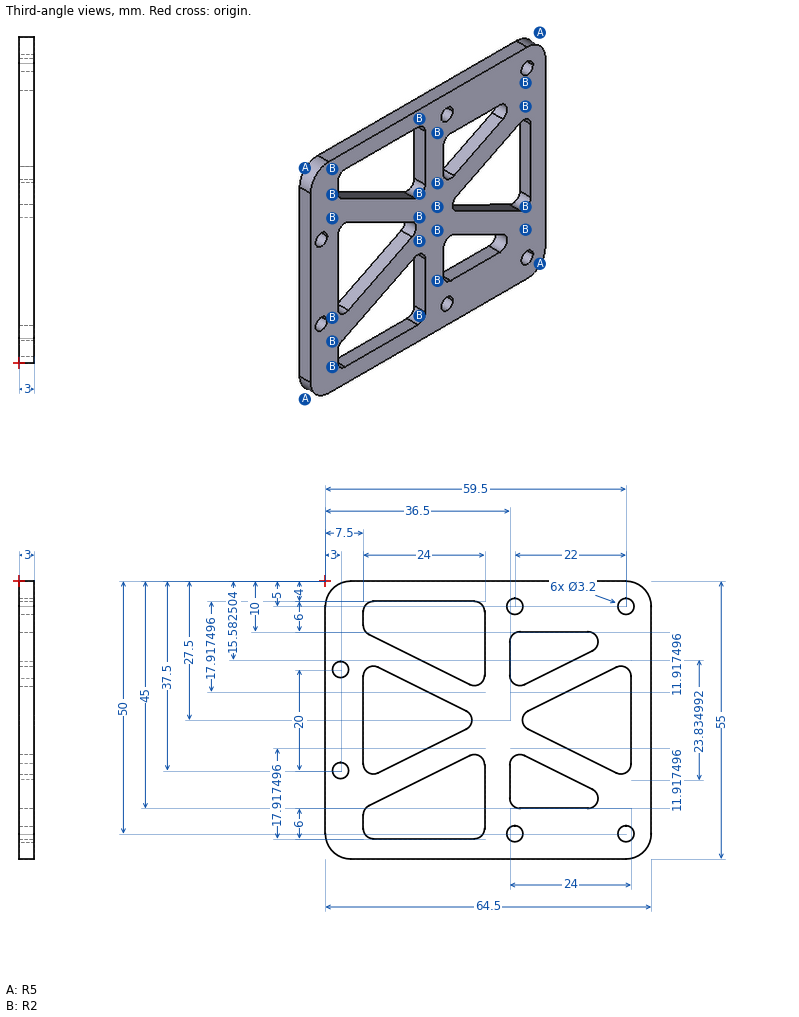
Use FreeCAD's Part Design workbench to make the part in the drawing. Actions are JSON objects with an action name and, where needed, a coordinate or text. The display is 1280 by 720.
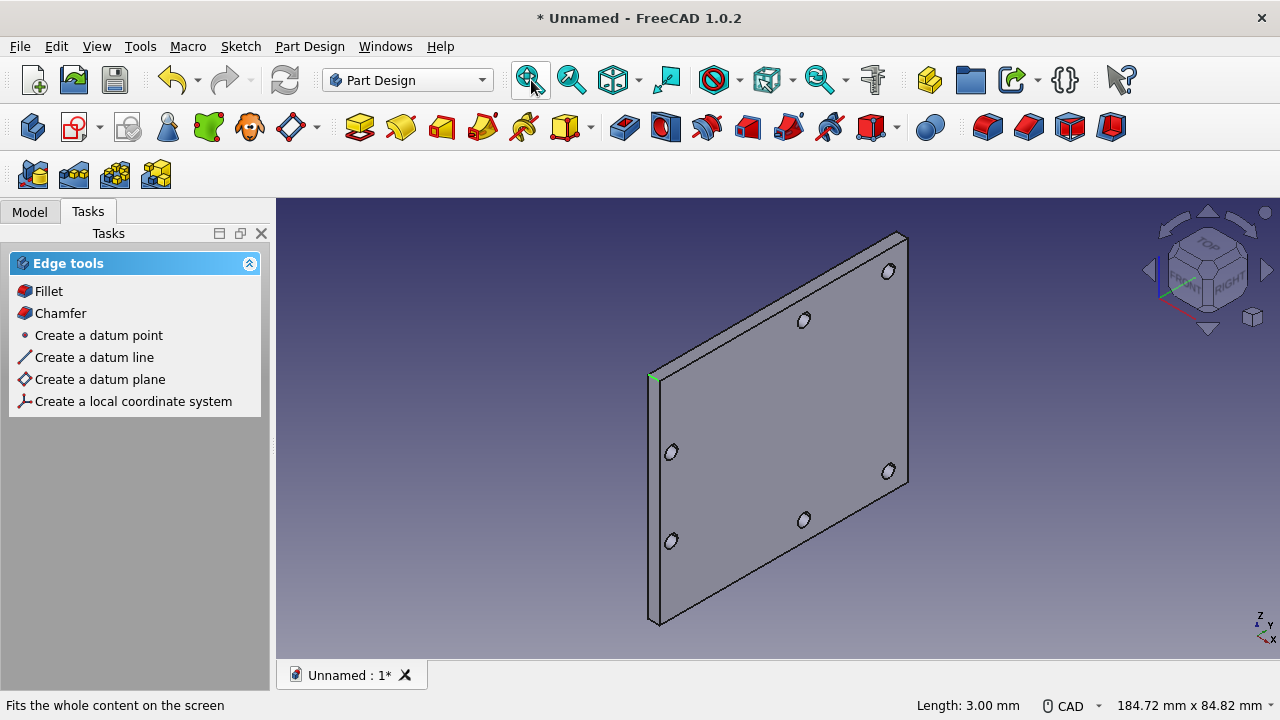
{"action": "scroll", "coordinate": [902, 234], "scroll_direction": "up", "scroll_amount": 5}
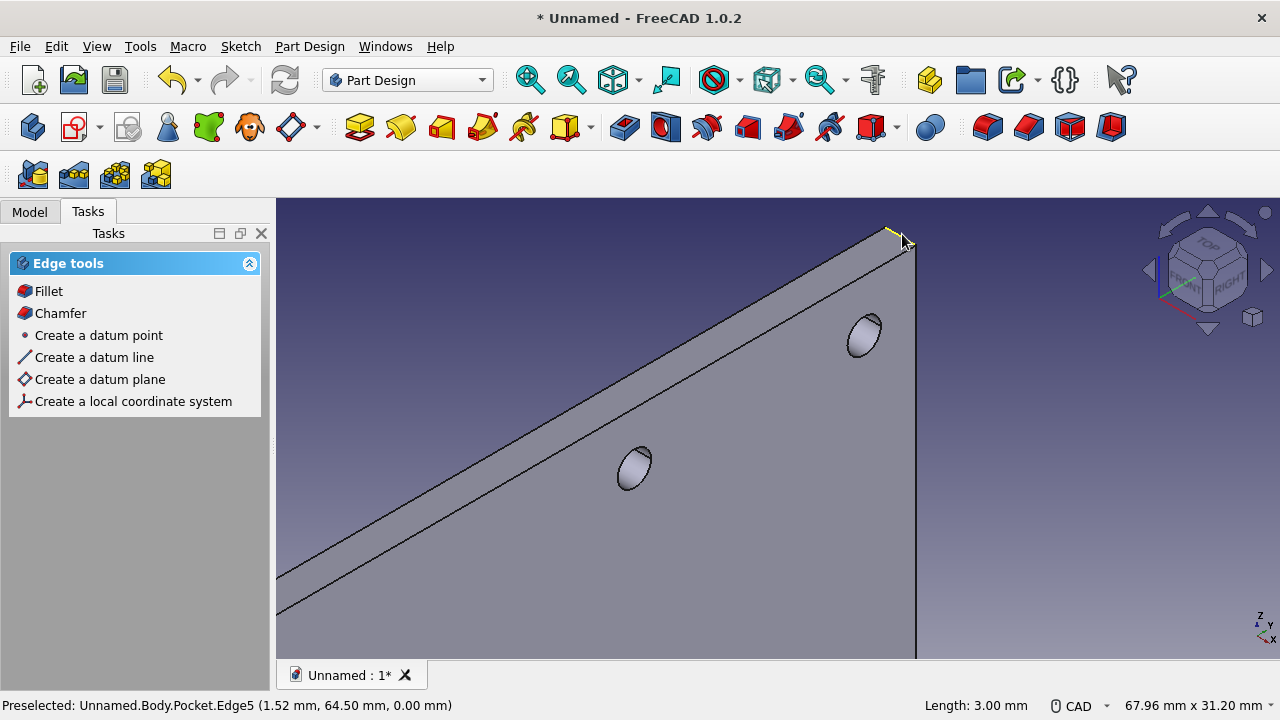
{"action": "left_click", "coordinate": [531, 80]}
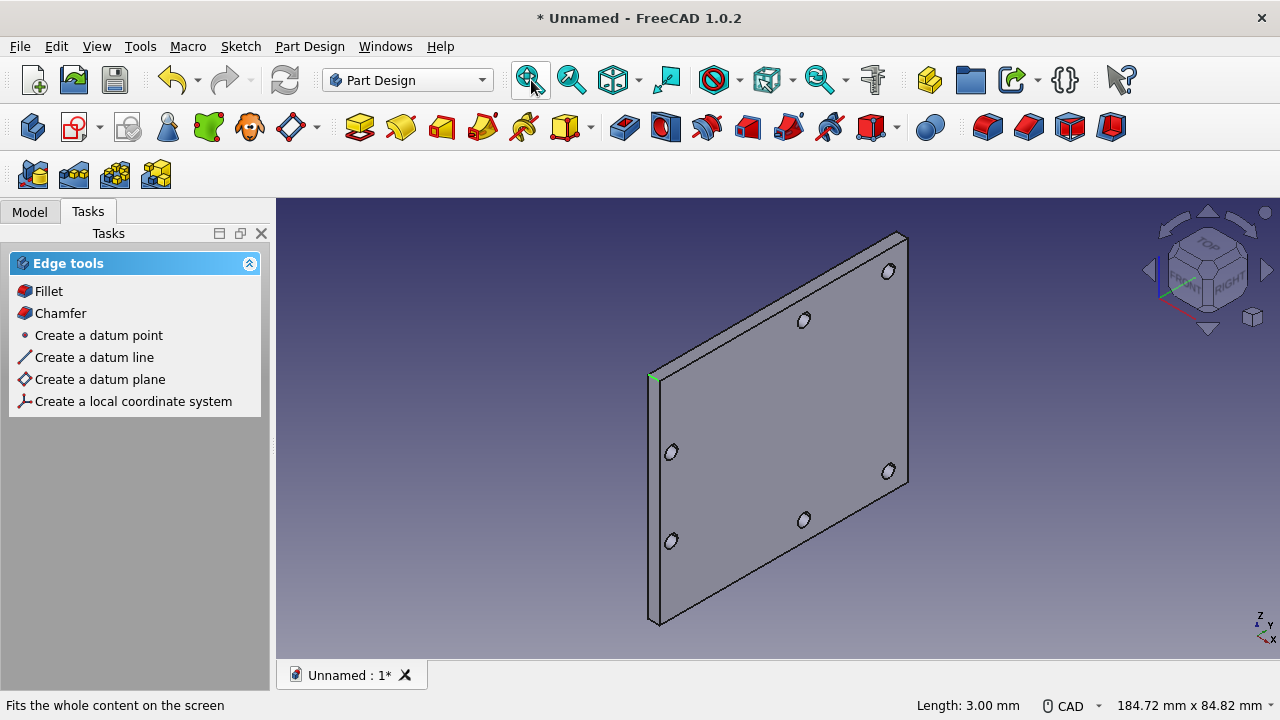
{"action": "key", "text": "2"}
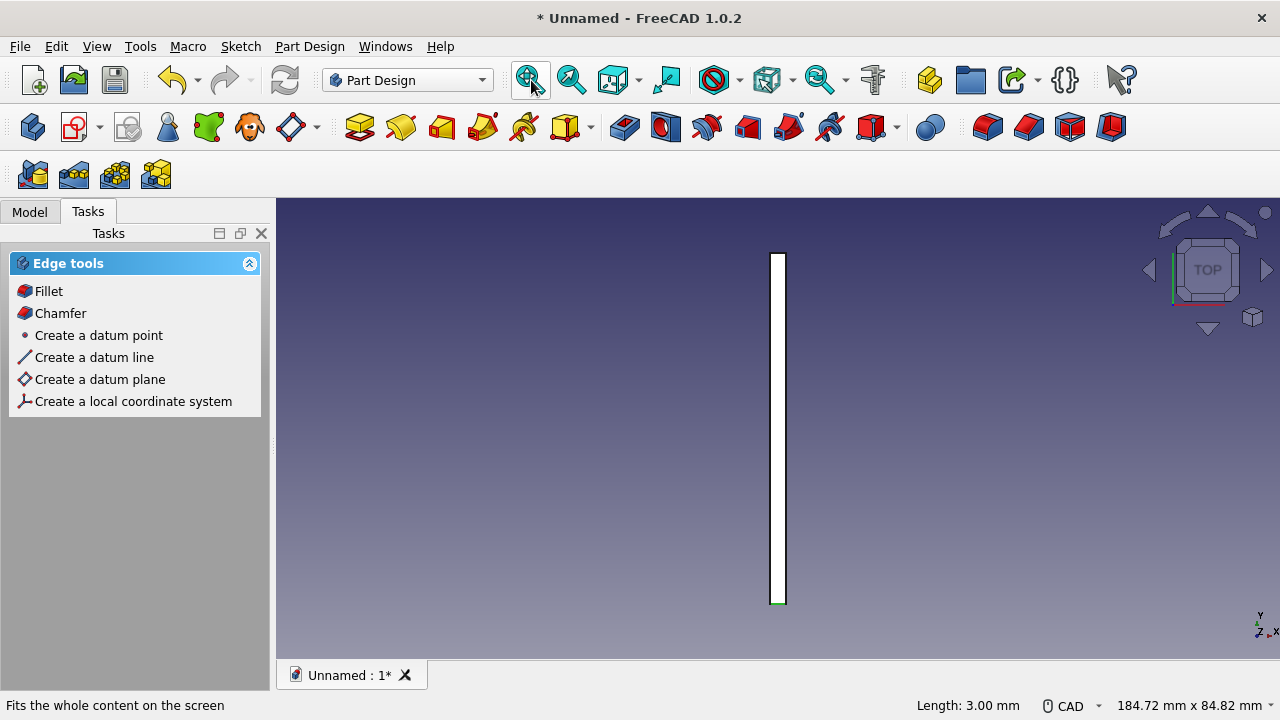
{"action": "scroll", "coordinate": [778, 252], "scroll_direction": "up", "scroll_amount": 5}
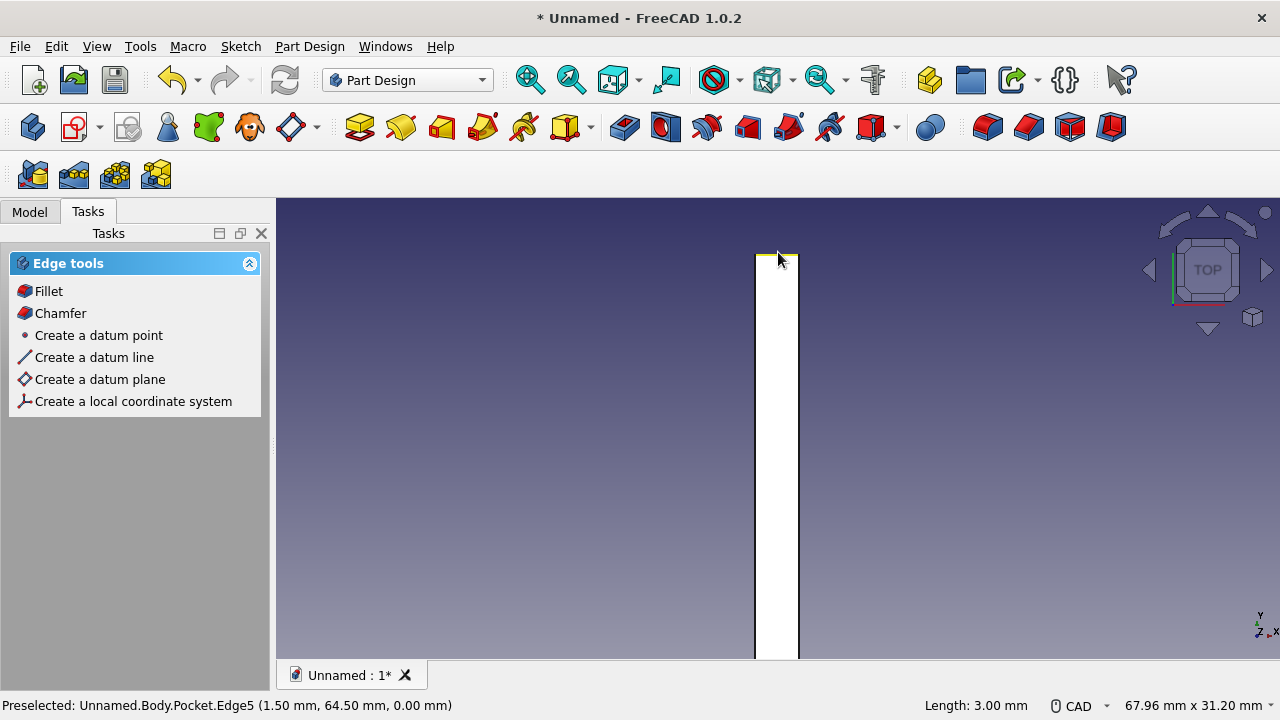
{"action": "left_click", "coordinate": [531, 80]}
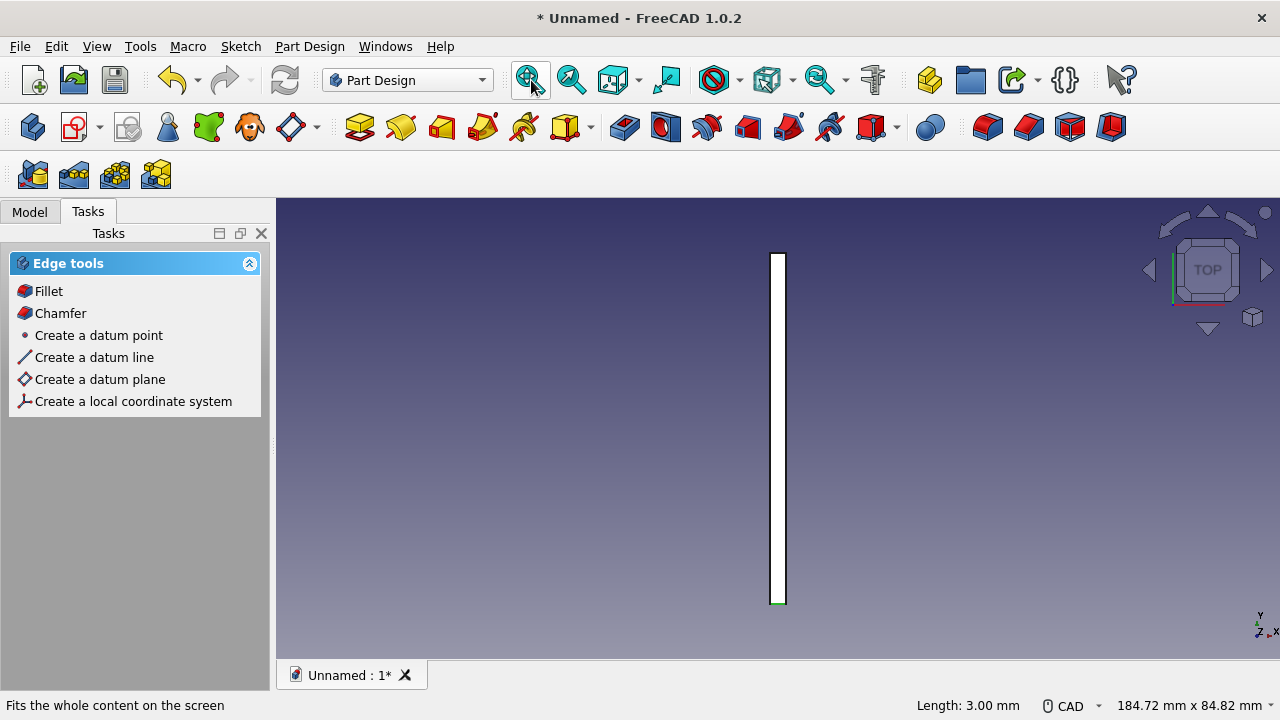
{"action": "key", "text": "1"}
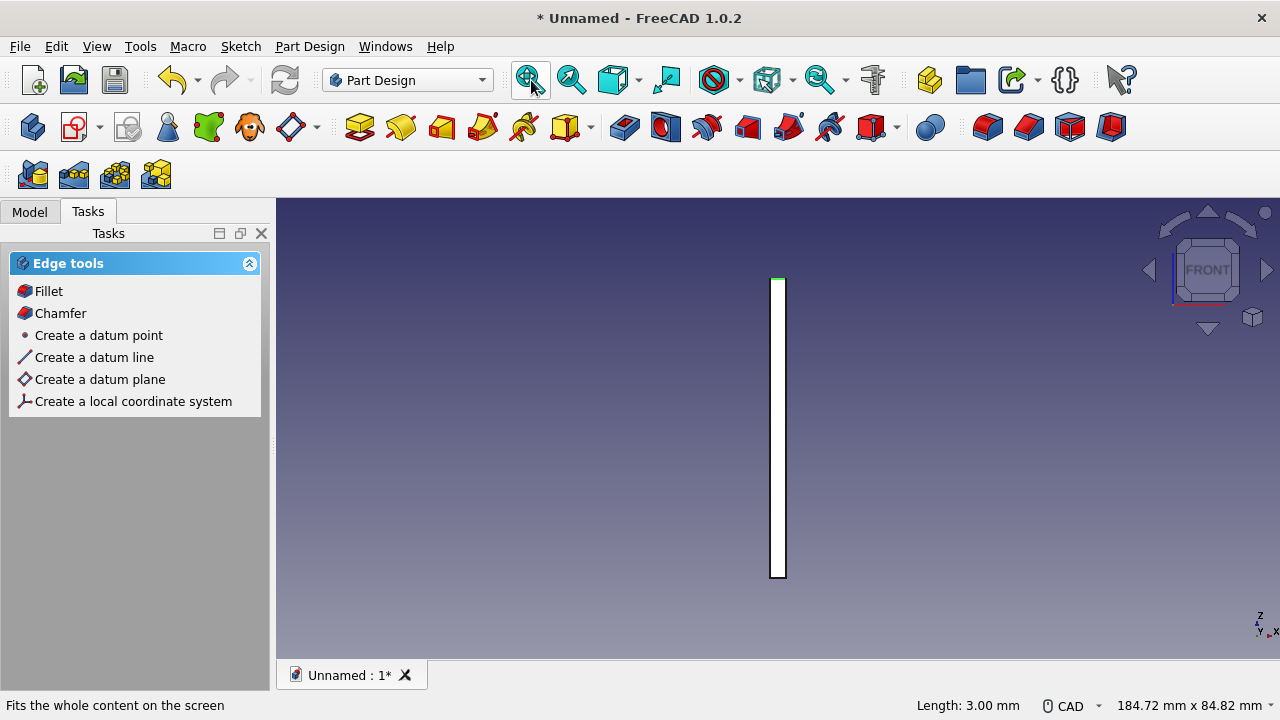
{"action": "left_click", "coordinate": [778, 577], "text": "ctrl"}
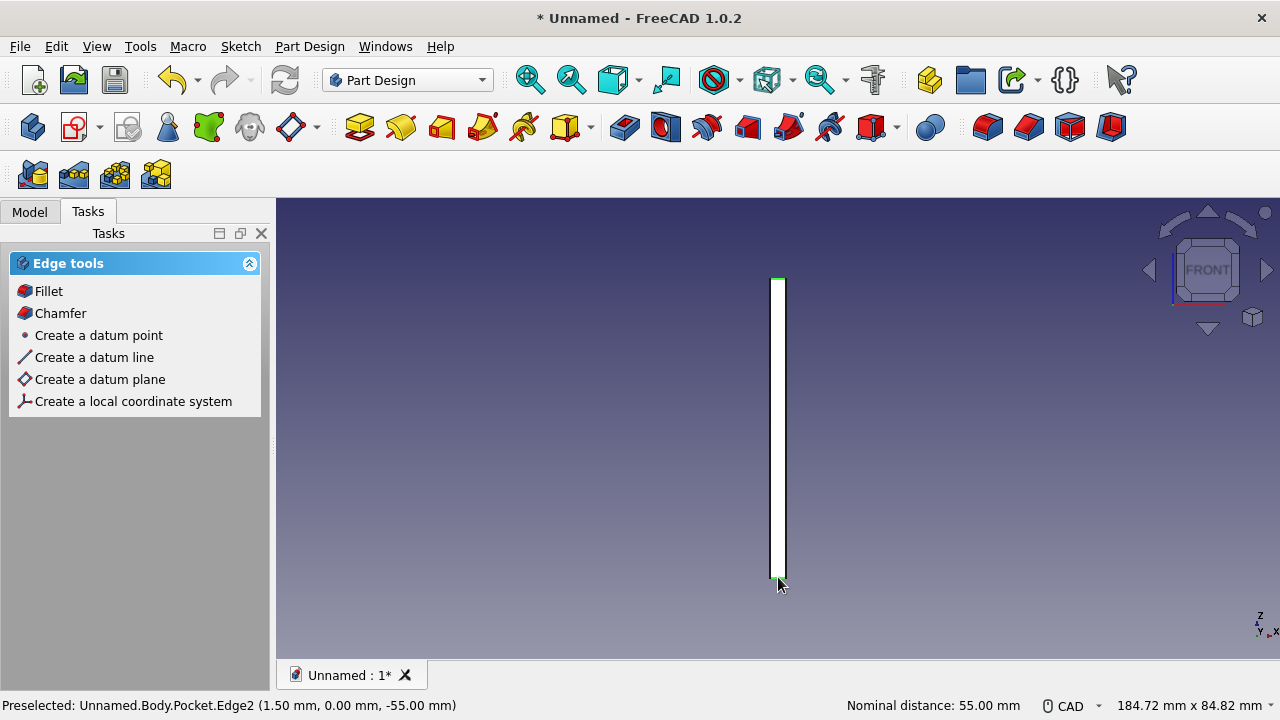
{"action": "scroll", "coordinate": [778, 278], "scroll_direction": "up", "scroll_amount": 5}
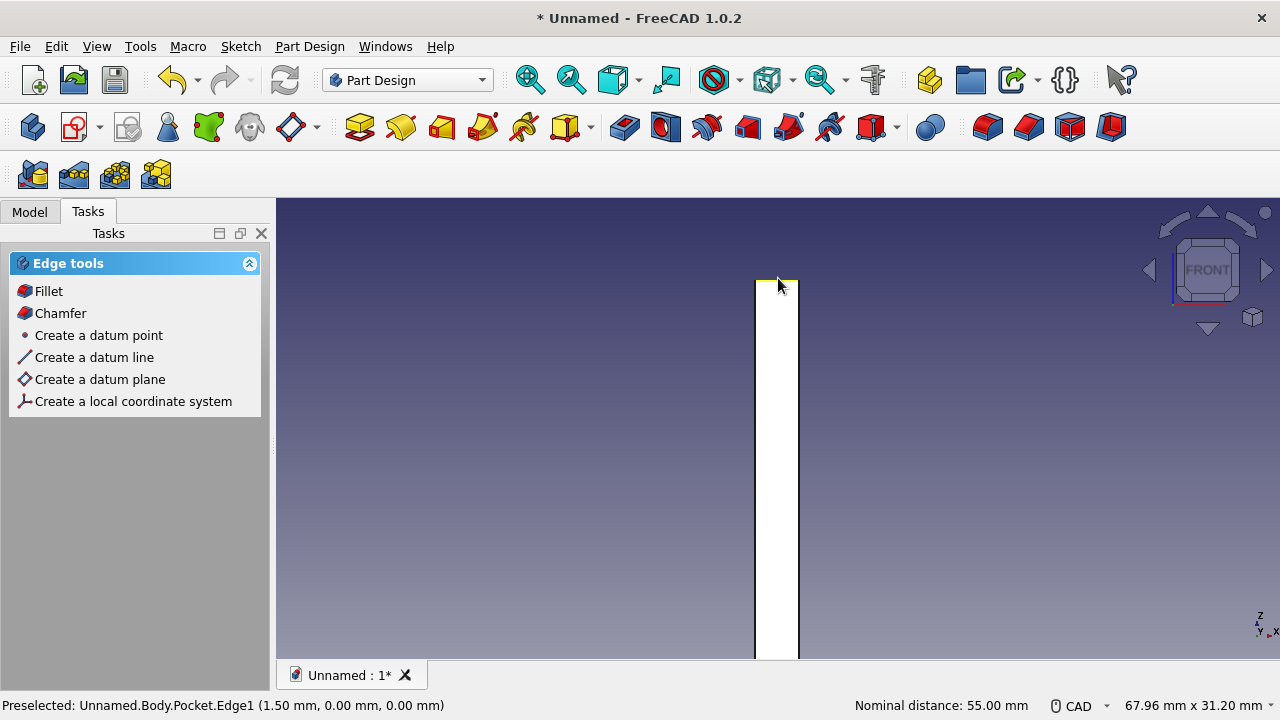
{"action": "key", "text": "v f"}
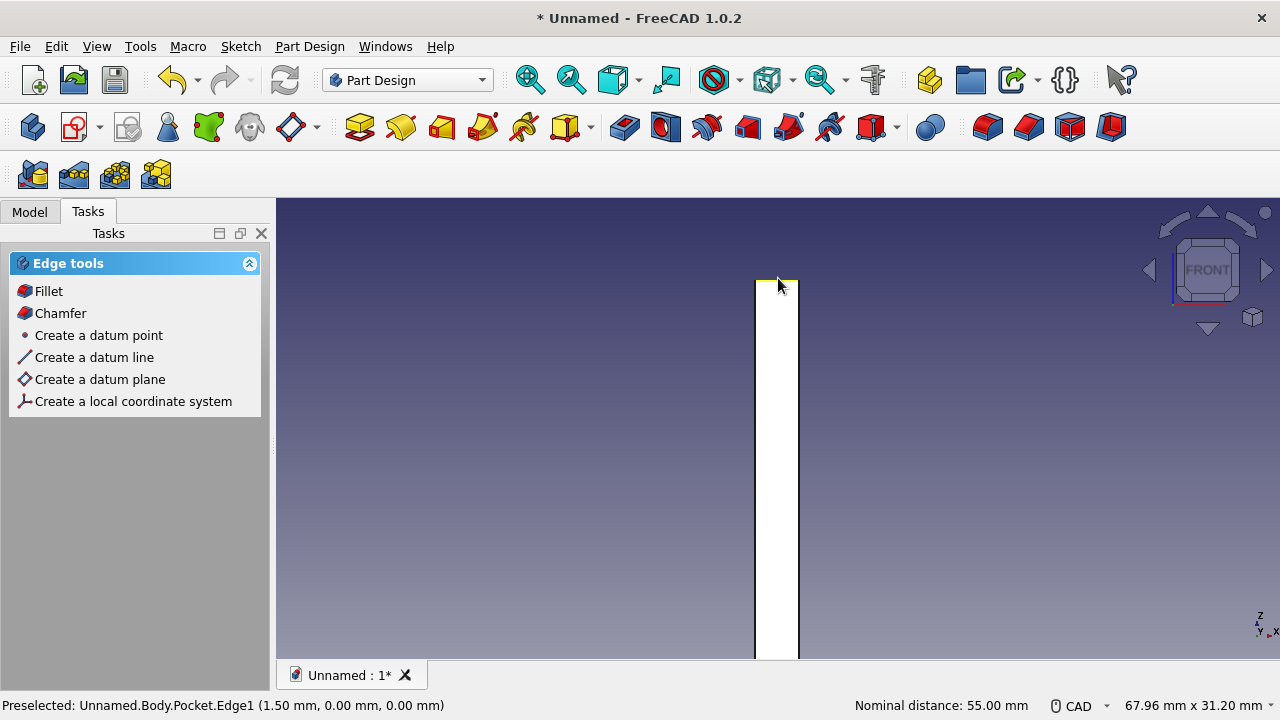
{"action": "key", "text": "3"}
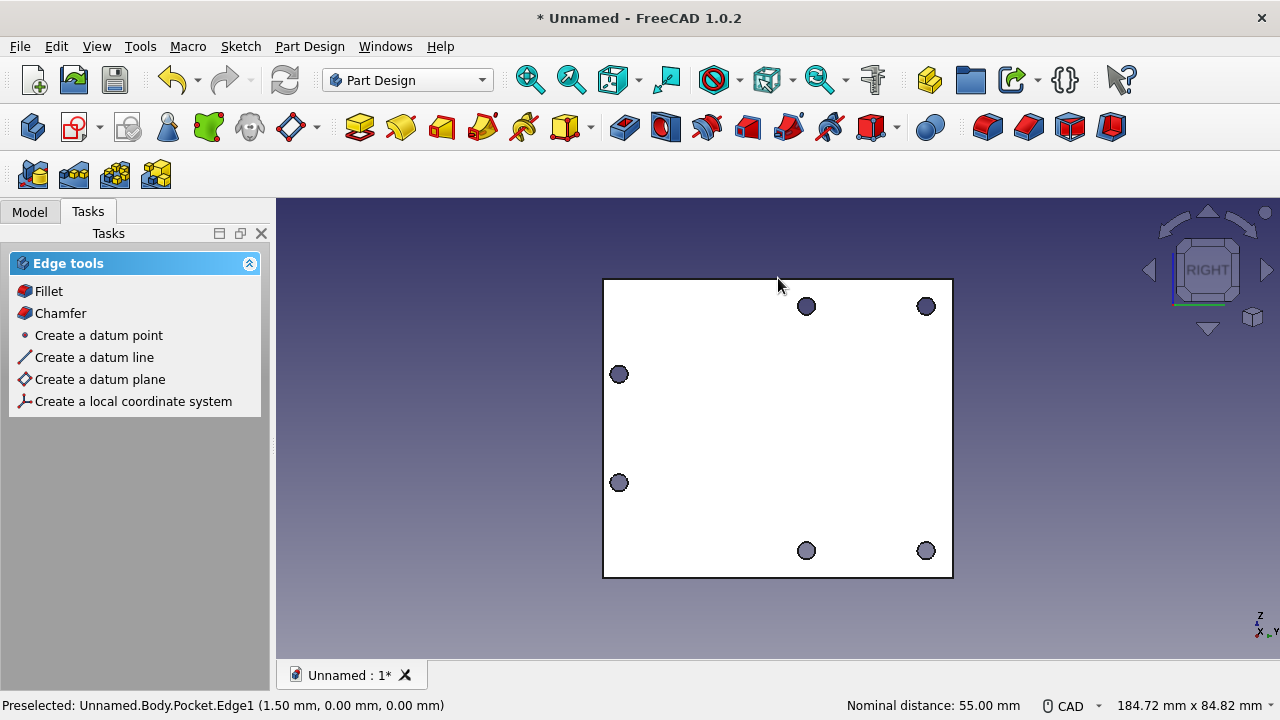
{"action": "scroll", "coordinate": [953, 278], "scroll_direction": "up", "scroll_amount": 5}